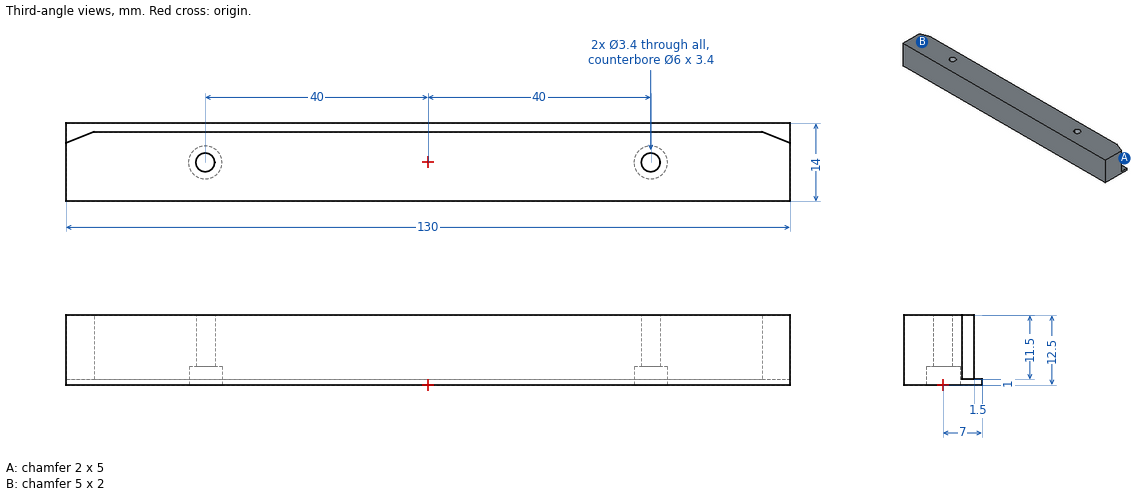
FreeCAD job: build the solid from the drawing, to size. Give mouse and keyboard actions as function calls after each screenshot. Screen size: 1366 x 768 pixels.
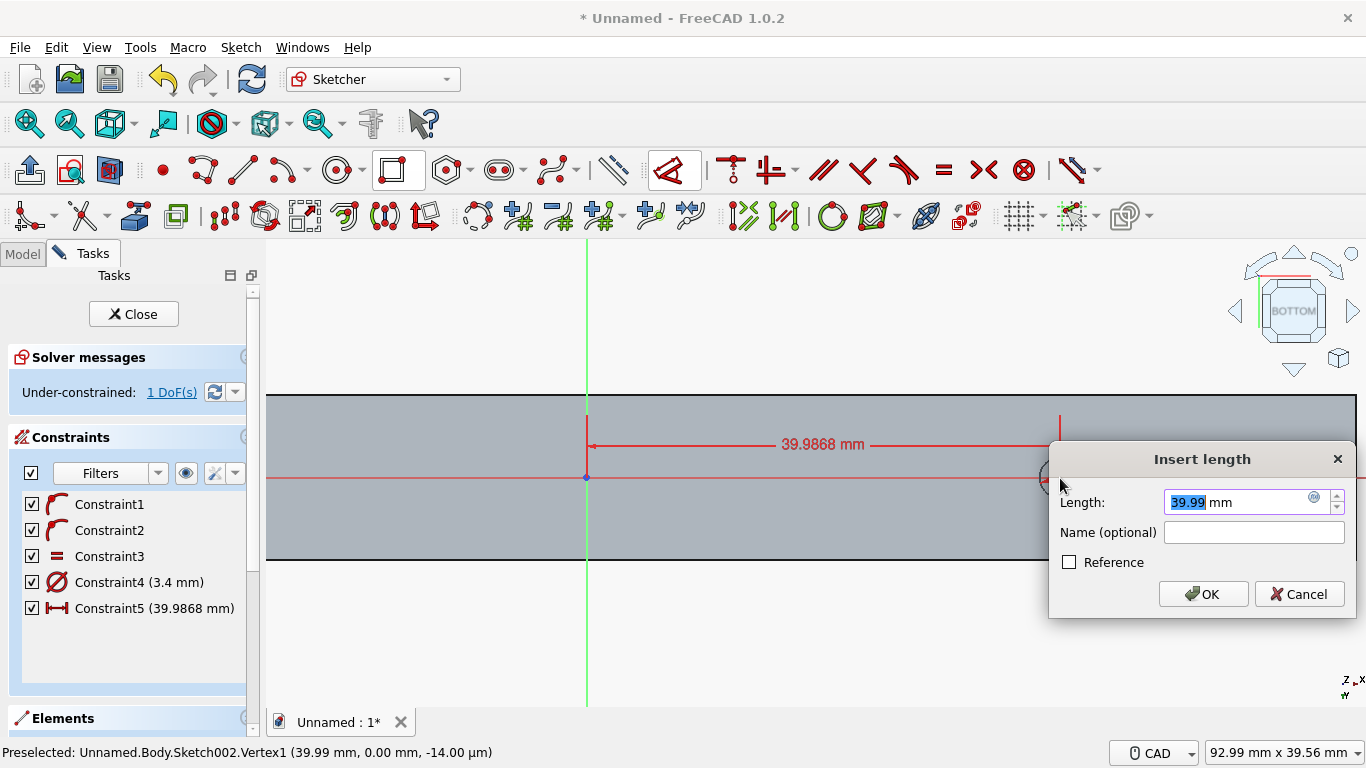
text(40)
key(Return)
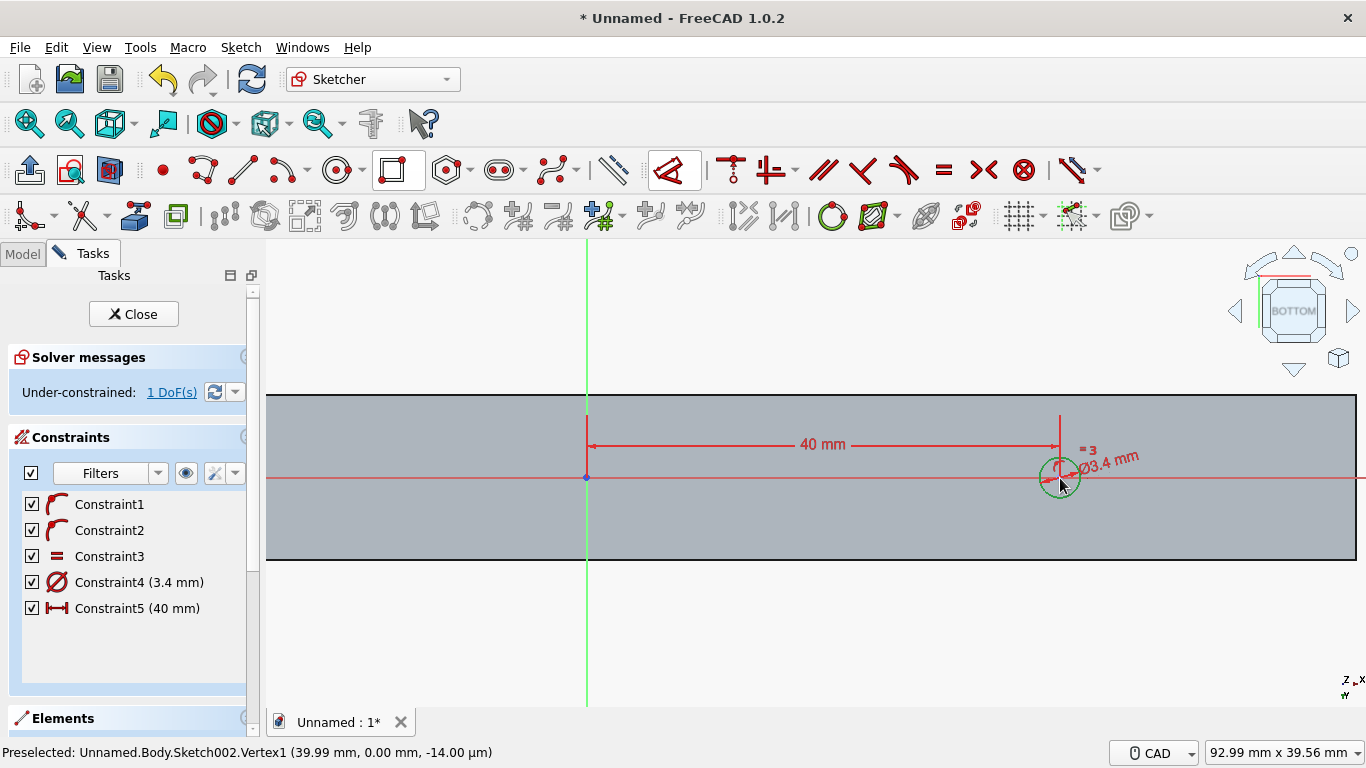
scroll(1074, 464, down, 2)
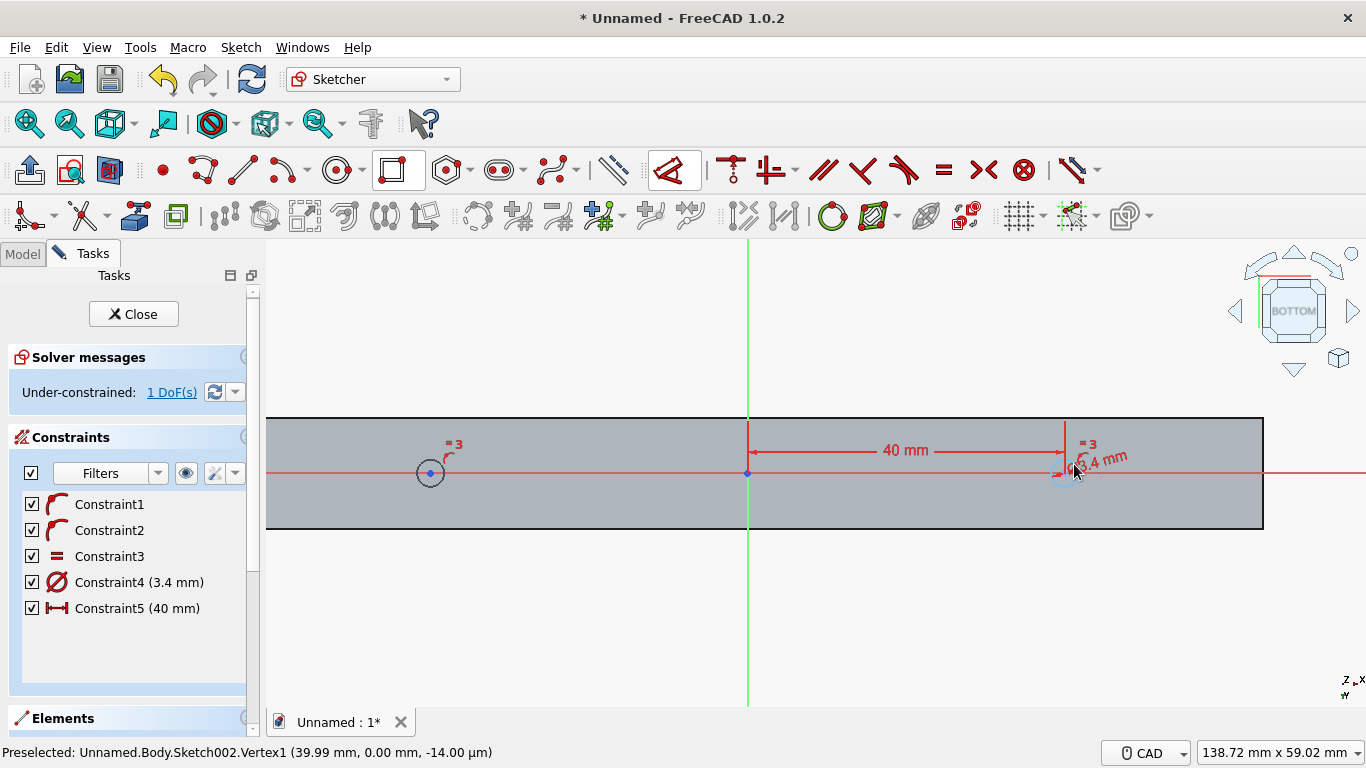
click(431, 473)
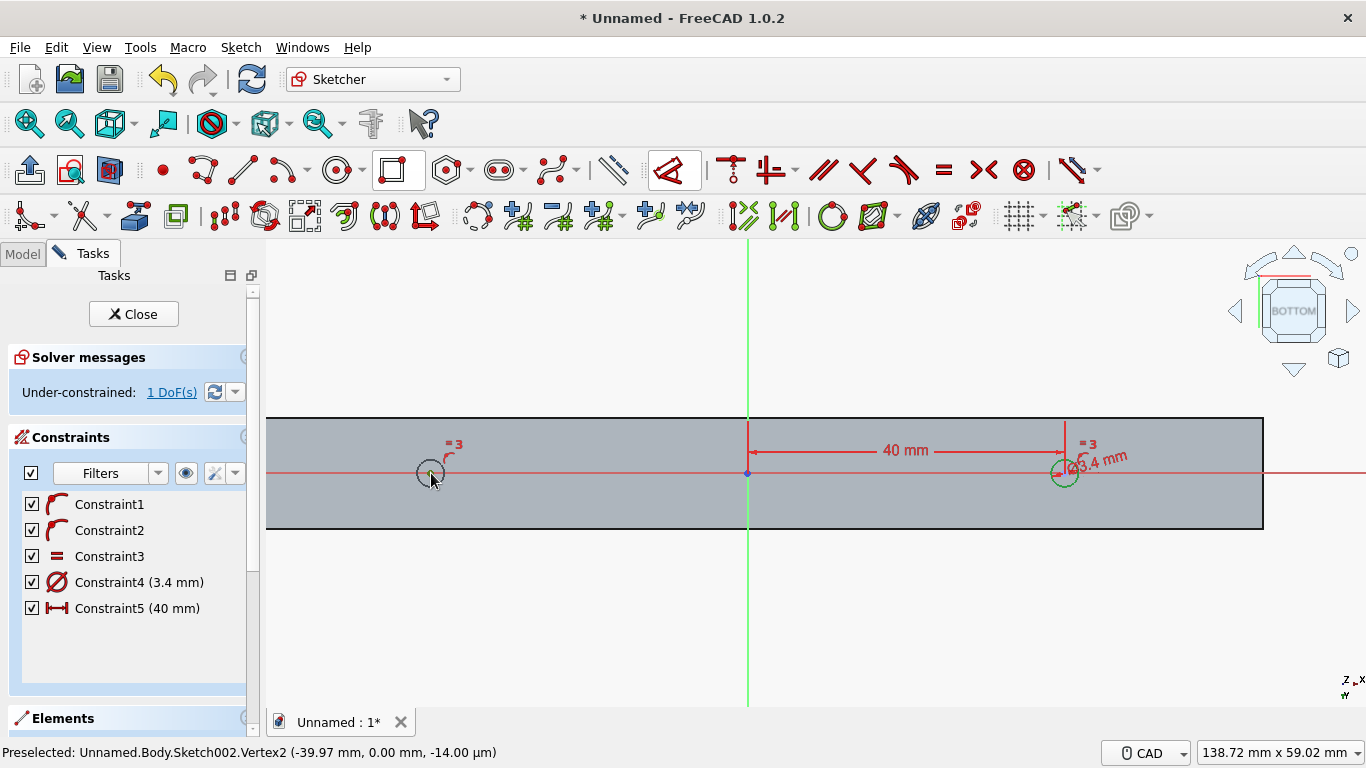
click(696, 170)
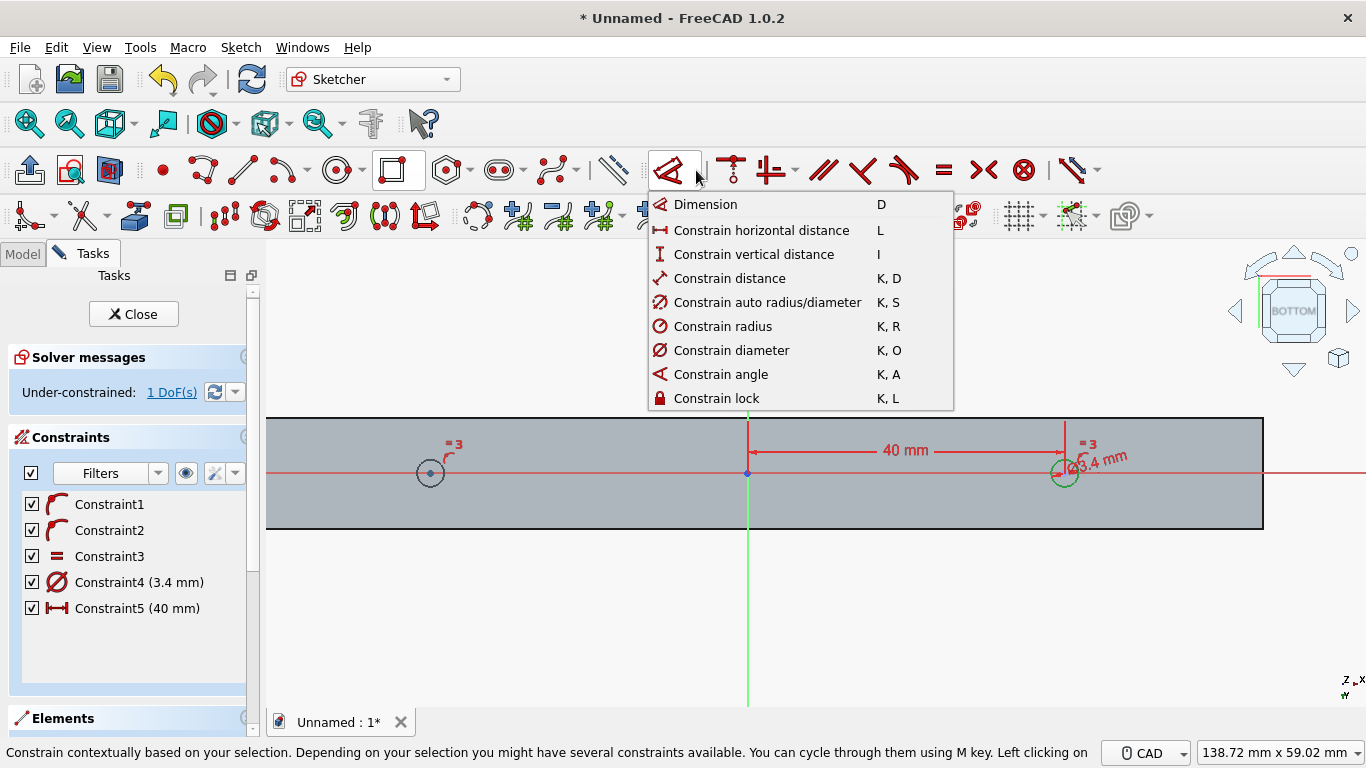
click(801, 230)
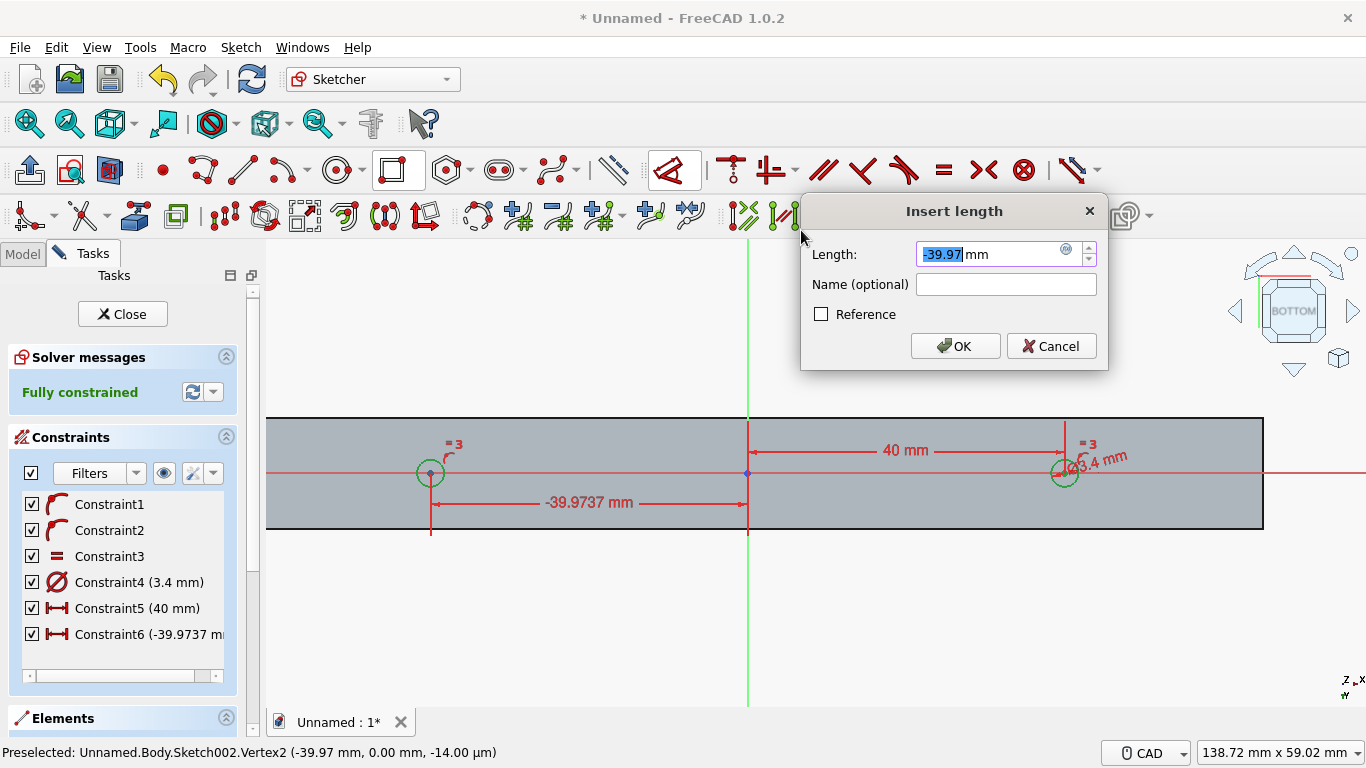
text(-40)
key(Return)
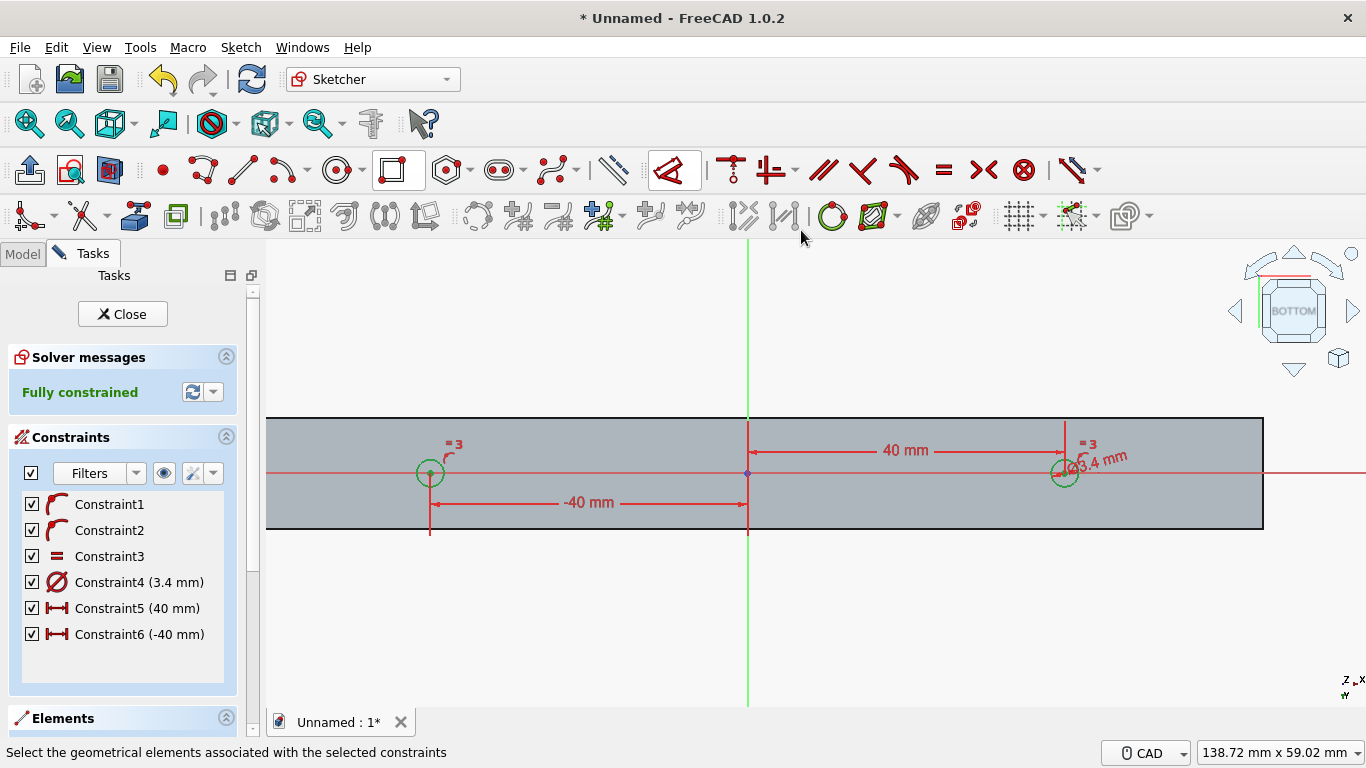
click(123, 314)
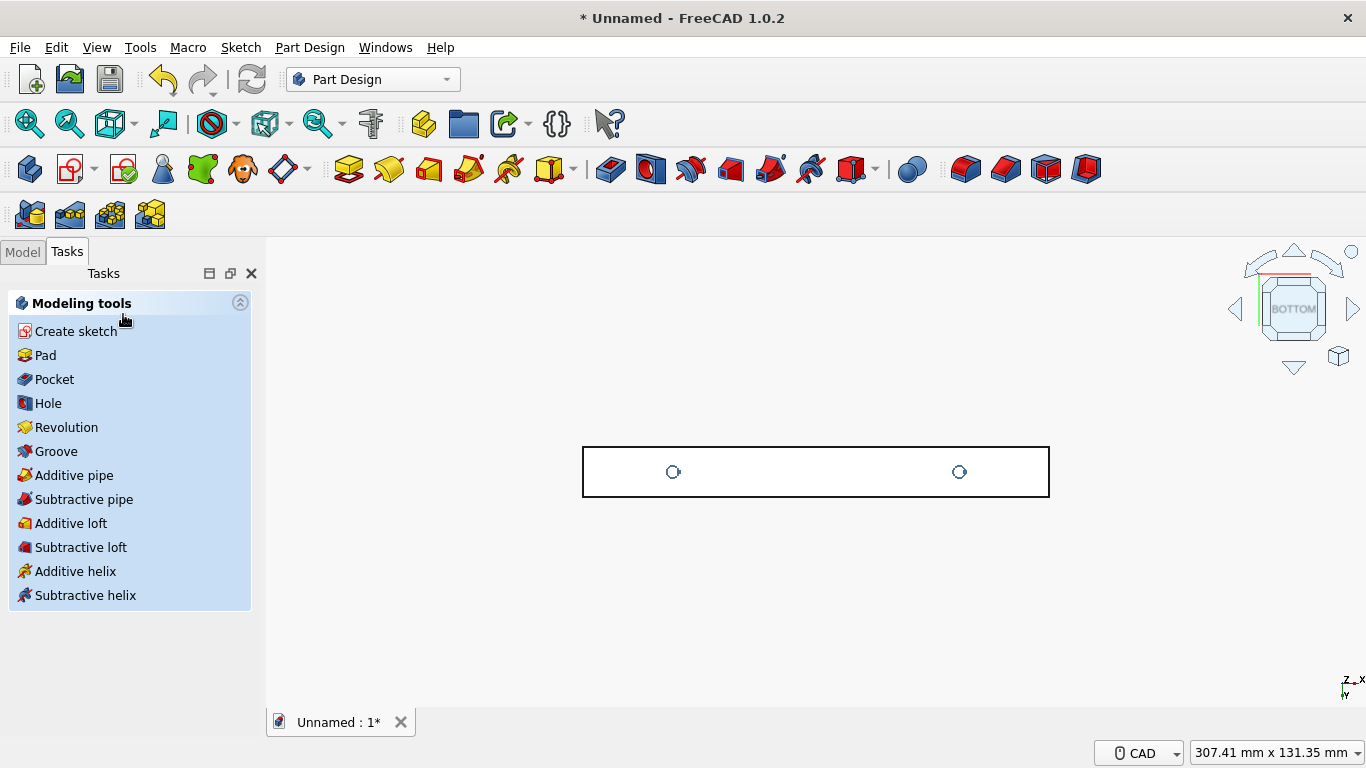
click(652, 170)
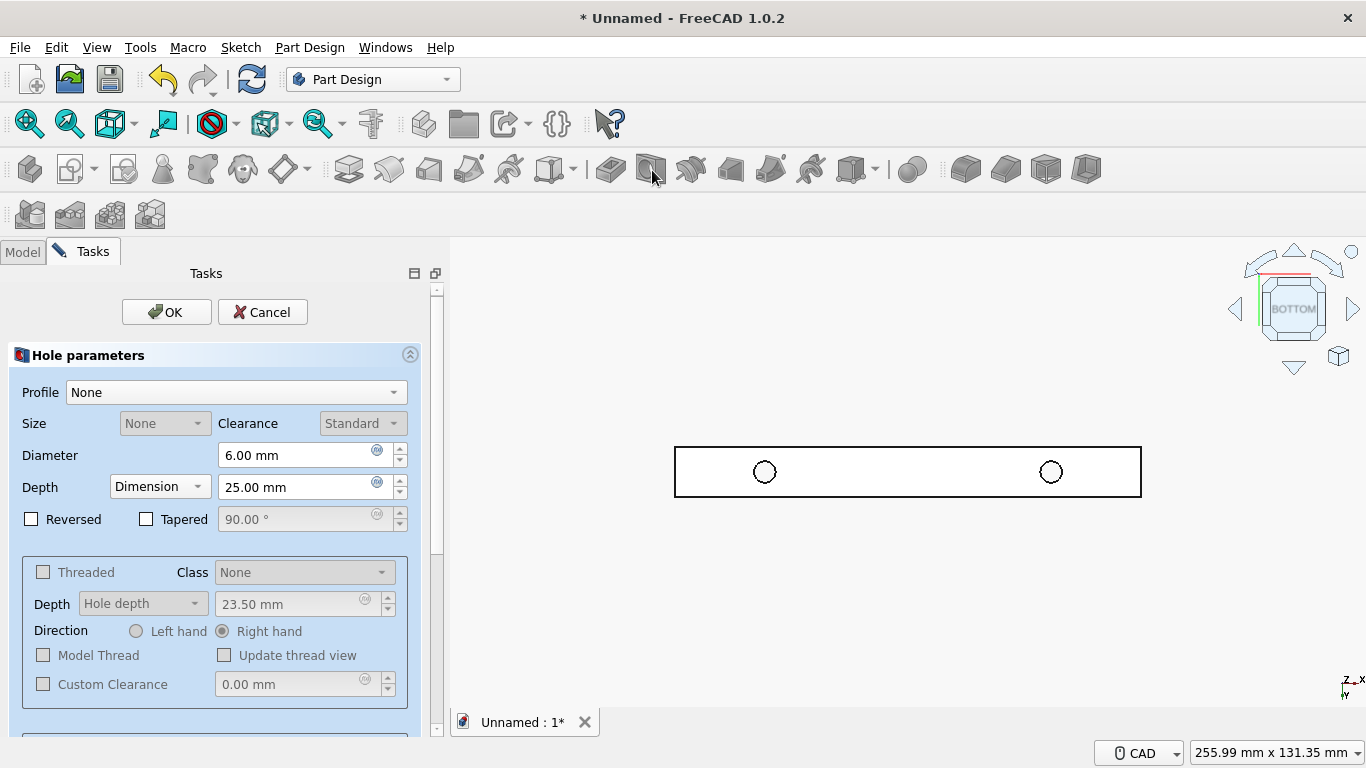
triple_click(305, 455)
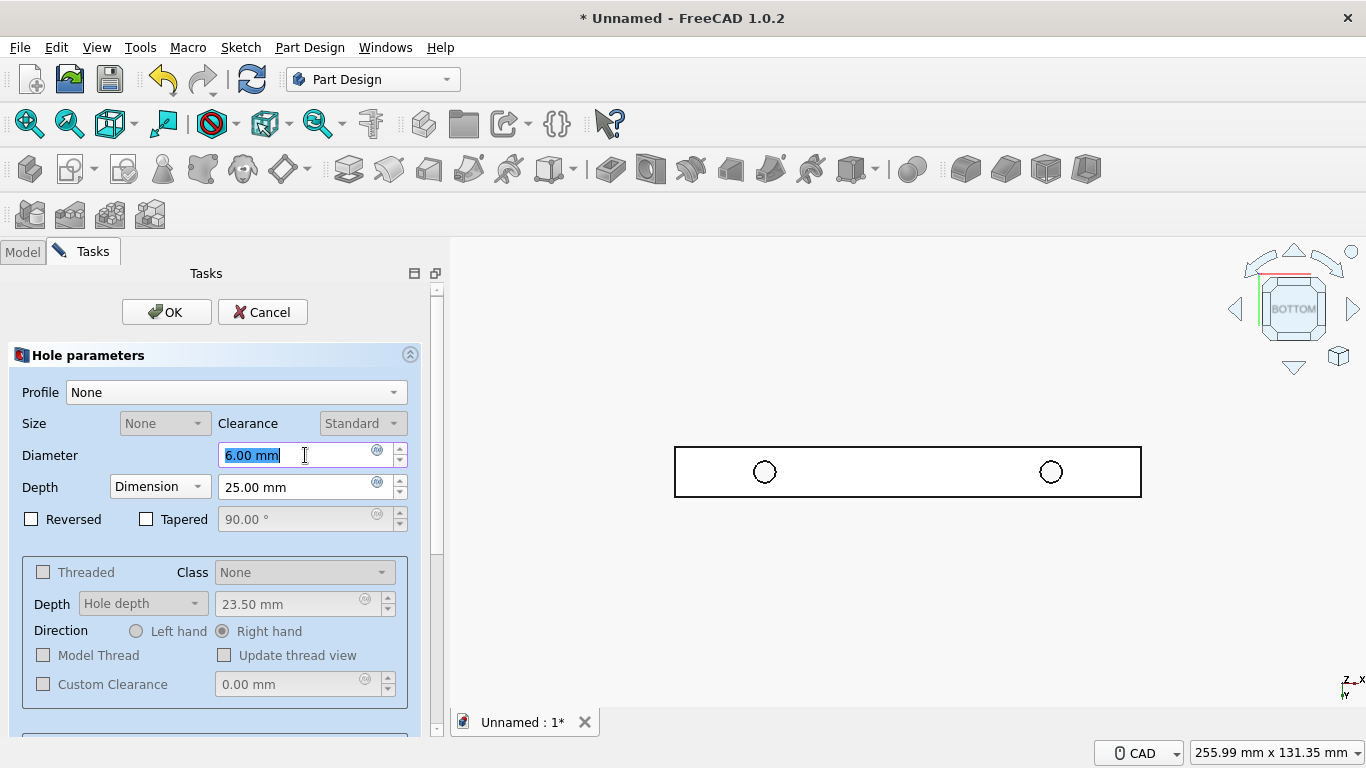
text(3.4)
key(Tab)